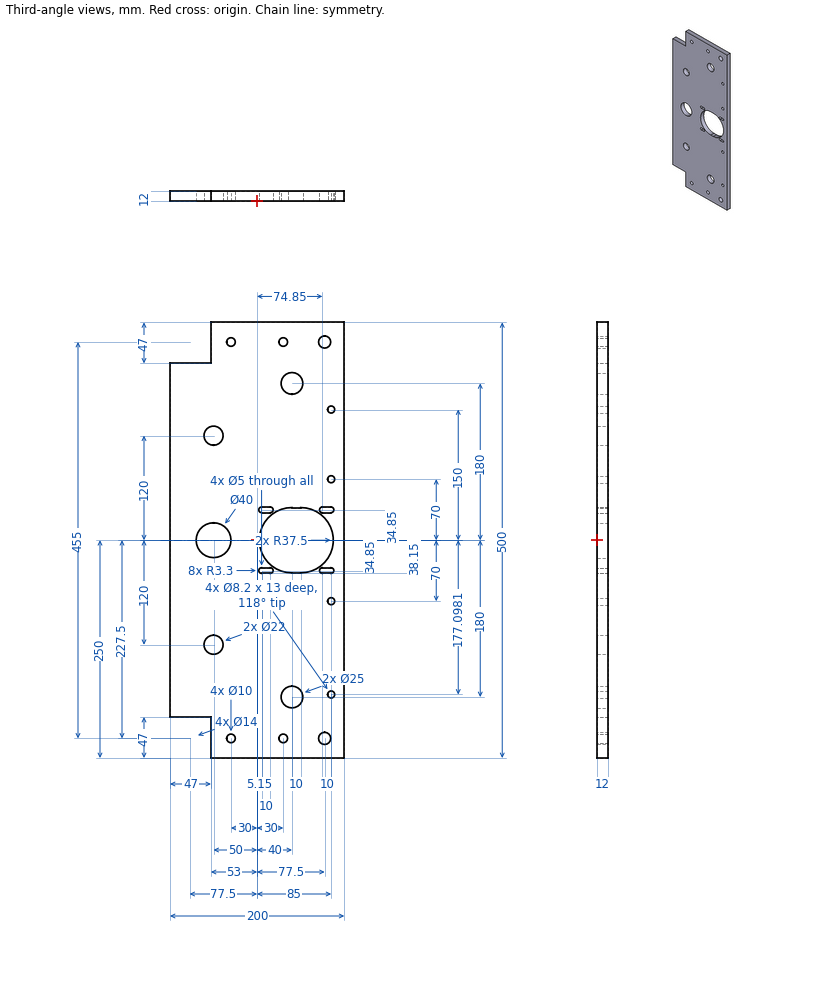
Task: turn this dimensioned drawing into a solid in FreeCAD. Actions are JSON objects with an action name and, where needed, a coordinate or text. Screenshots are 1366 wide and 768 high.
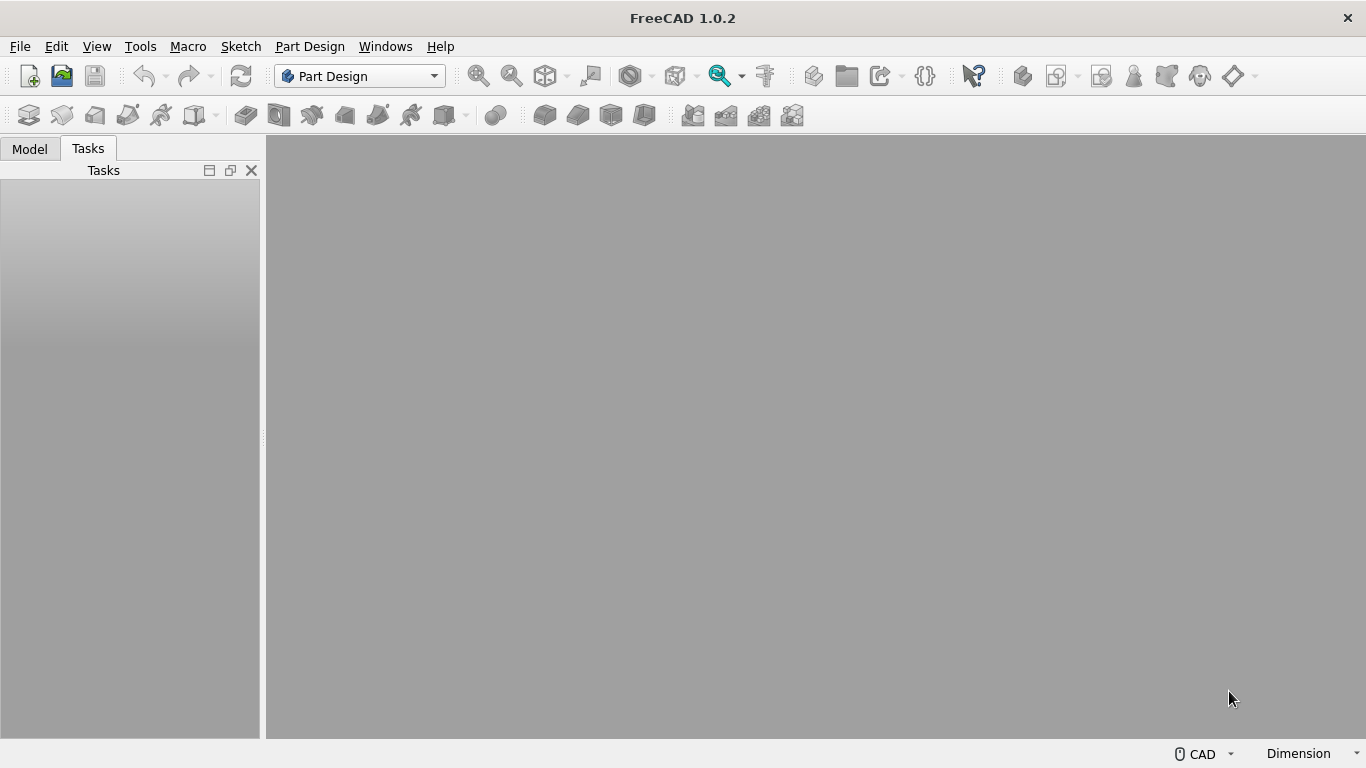
{"action": "key", "text": "ctrl+n"}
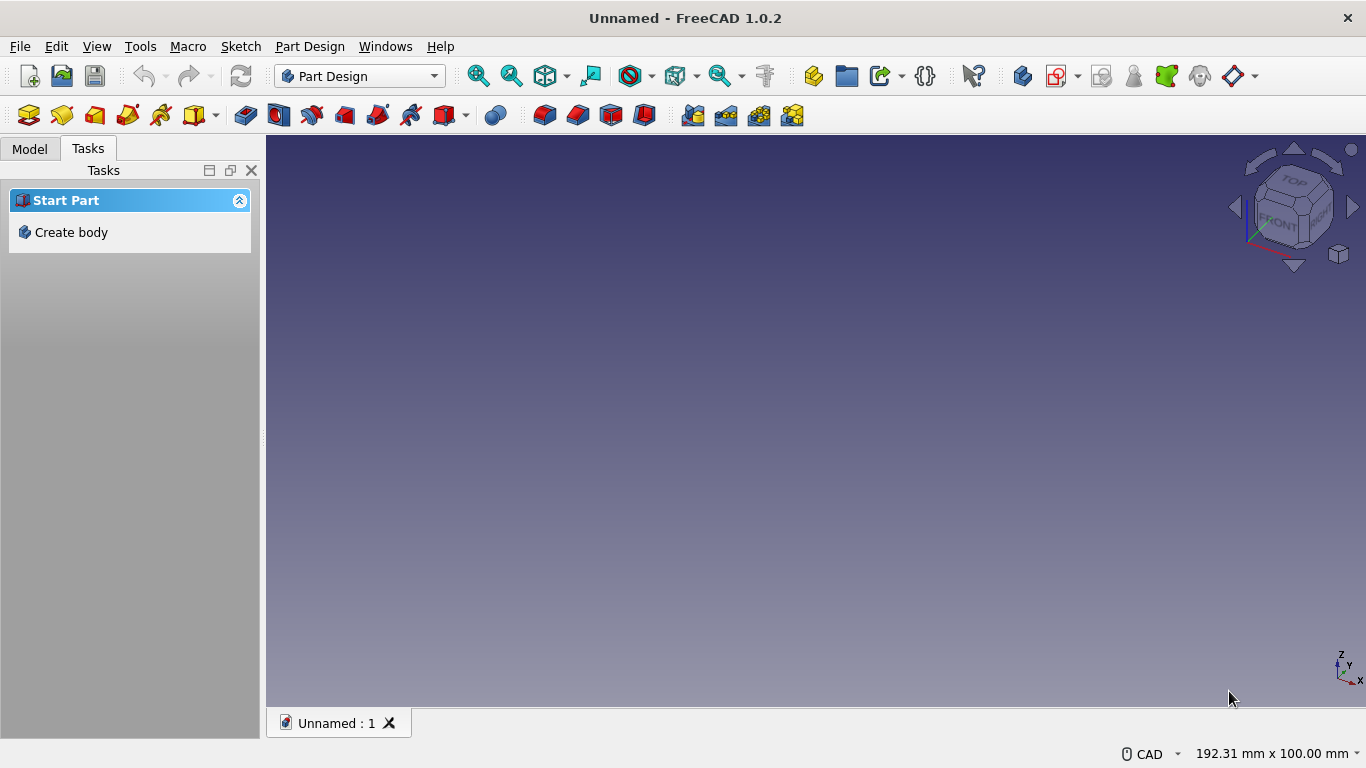
{"action": "left_click", "coordinate": [1056, 76]}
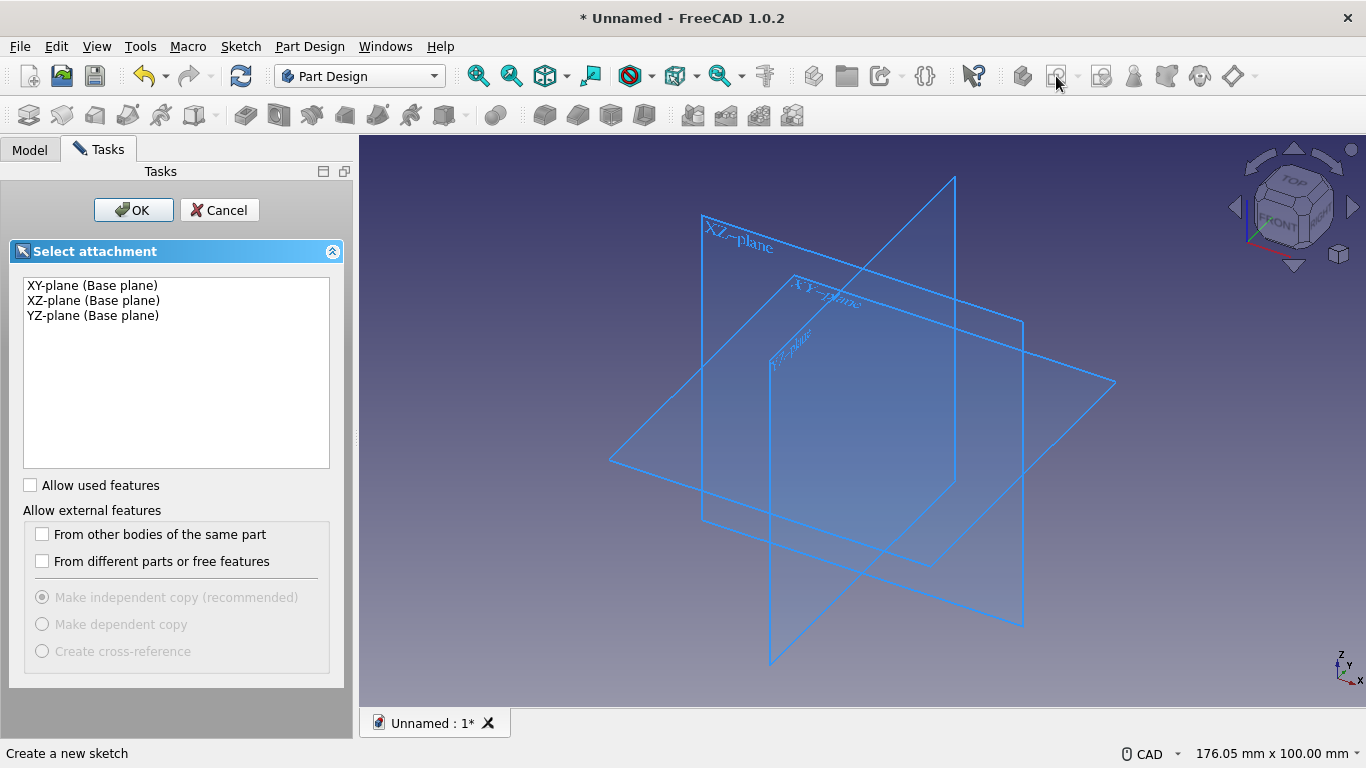
{"action": "left_click", "coordinate": [84, 300]}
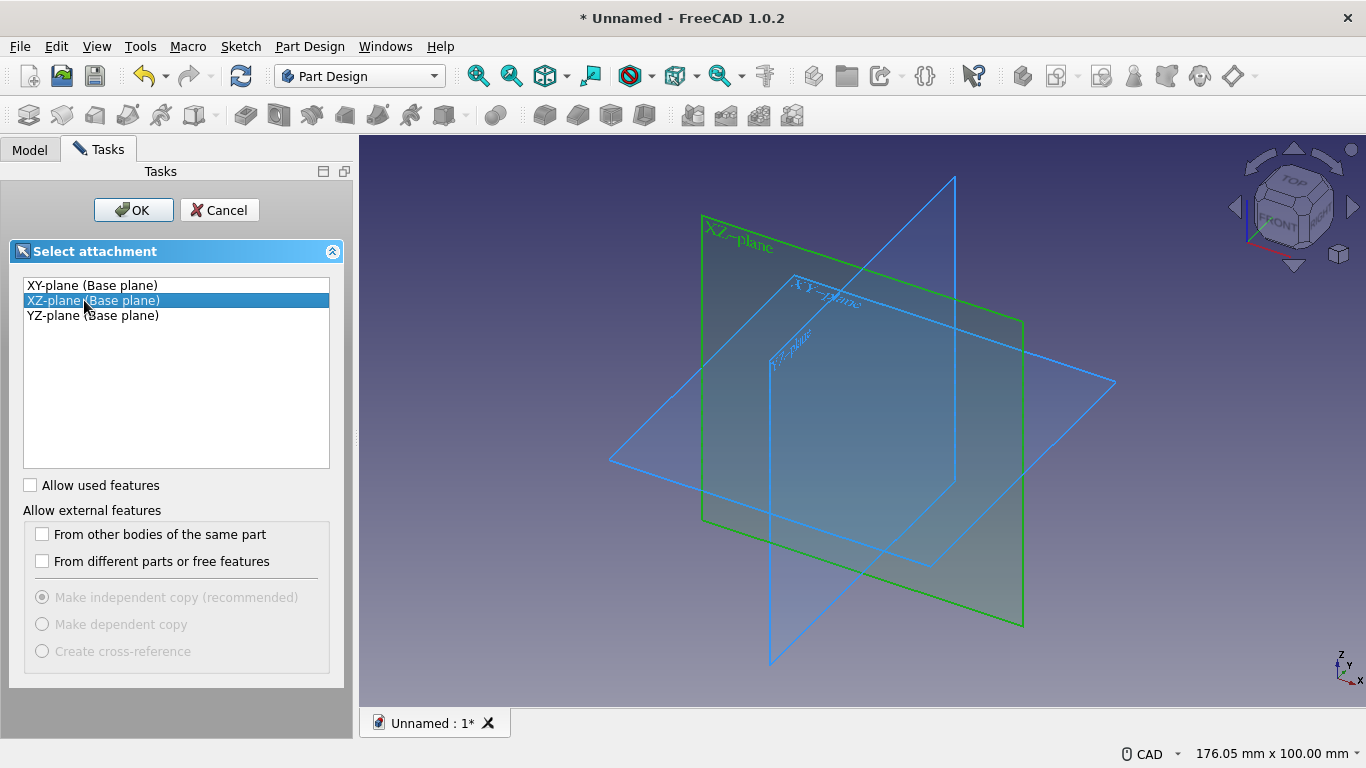
{"action": "left_click", "coordinate": [134, 210]}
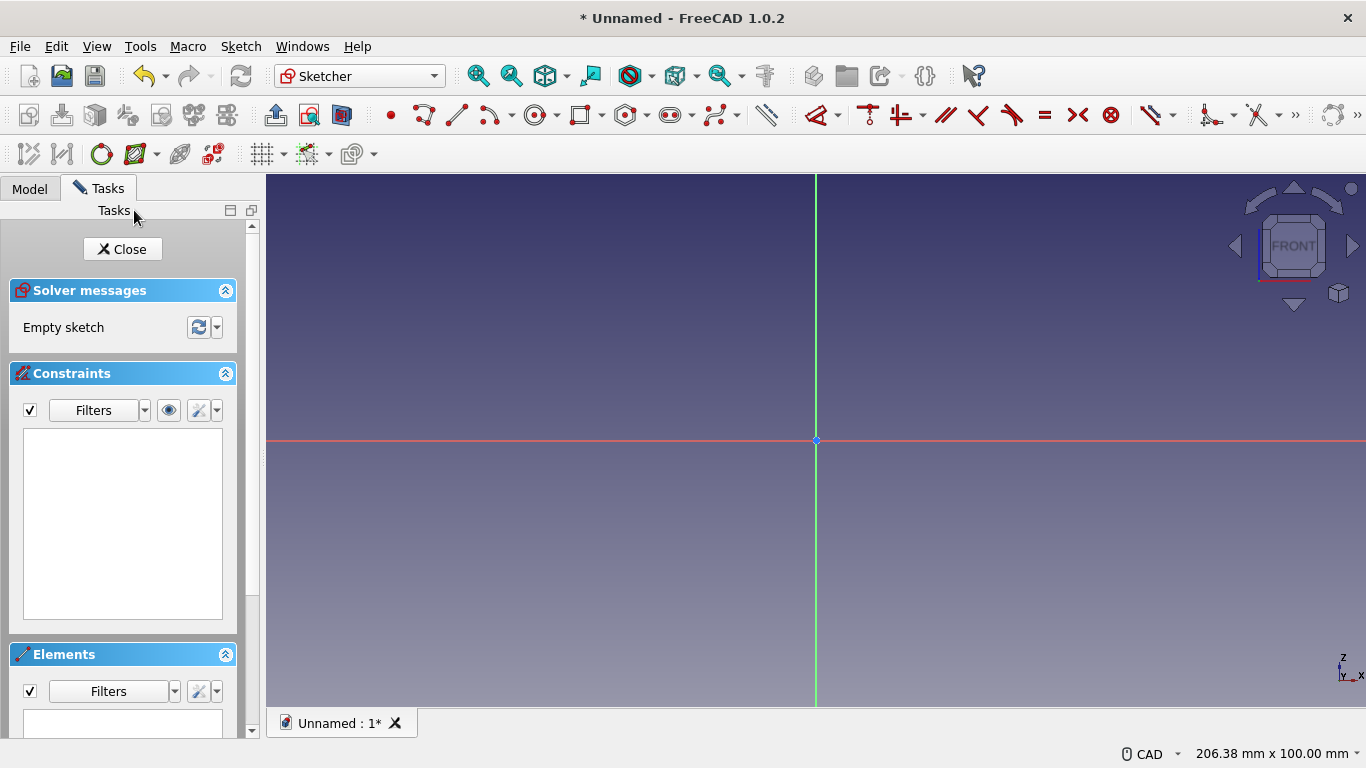
{"action": "scroll", "coordinate": [737, 440], "scroll_direction": "down", "scroll_amount": 10}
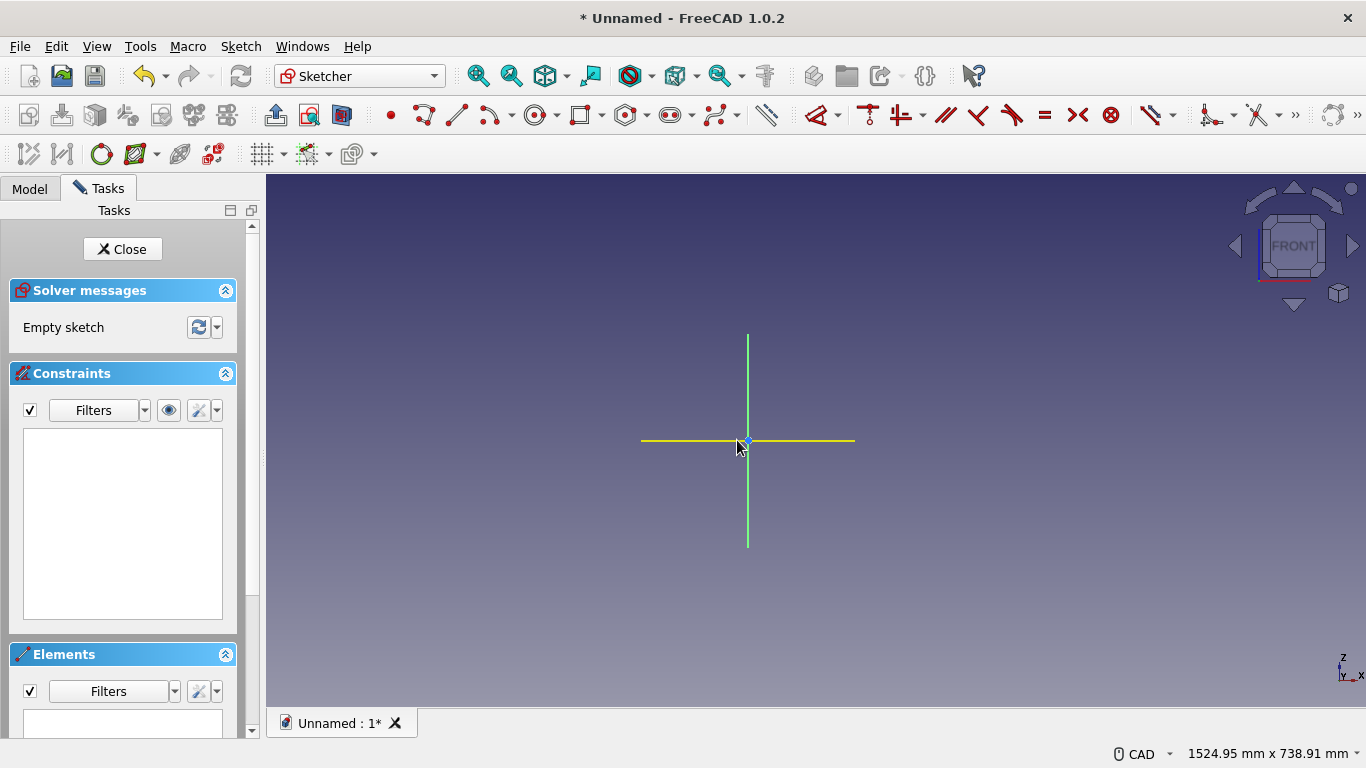
{"action": "key", "text": "g v"}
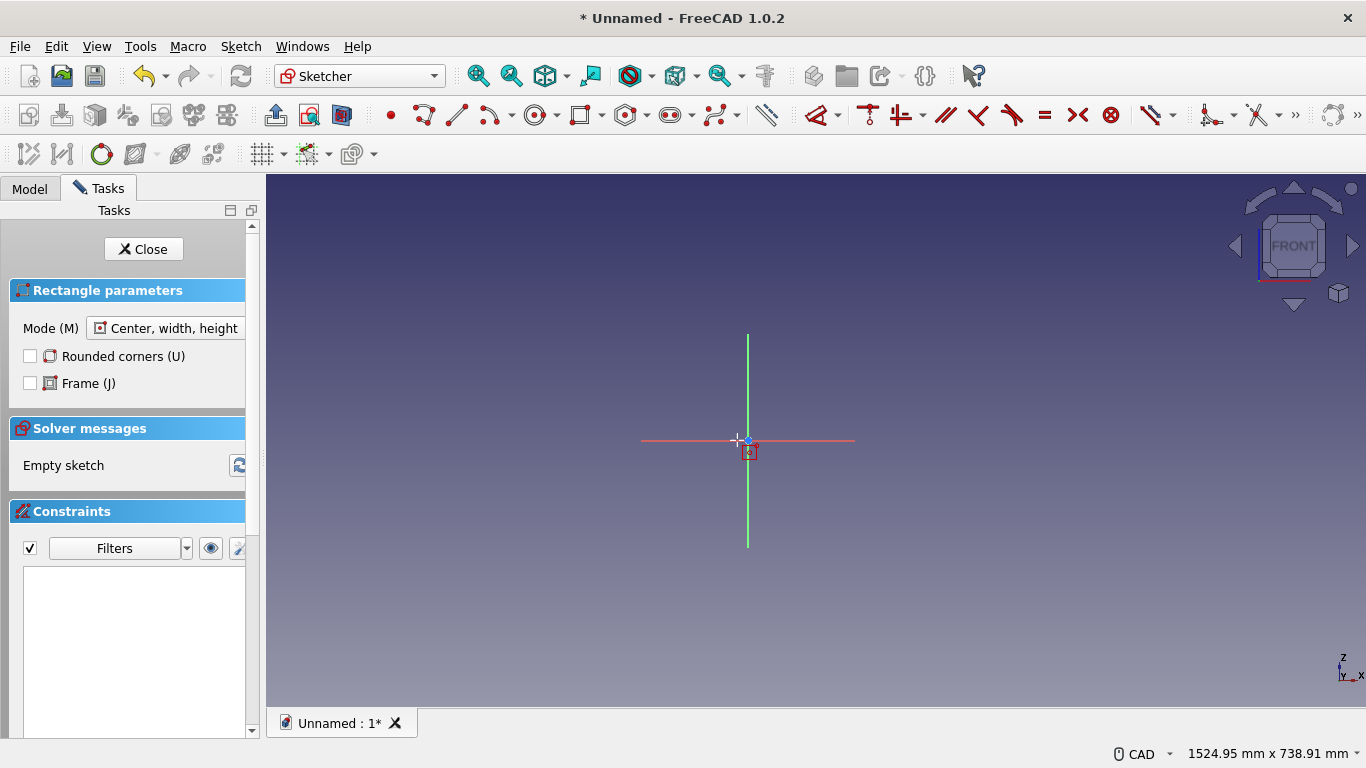
{"action": "left_click", "coordinate": [748, 440]}
{"action": "mouse_move", "coordinate": [820, 260]}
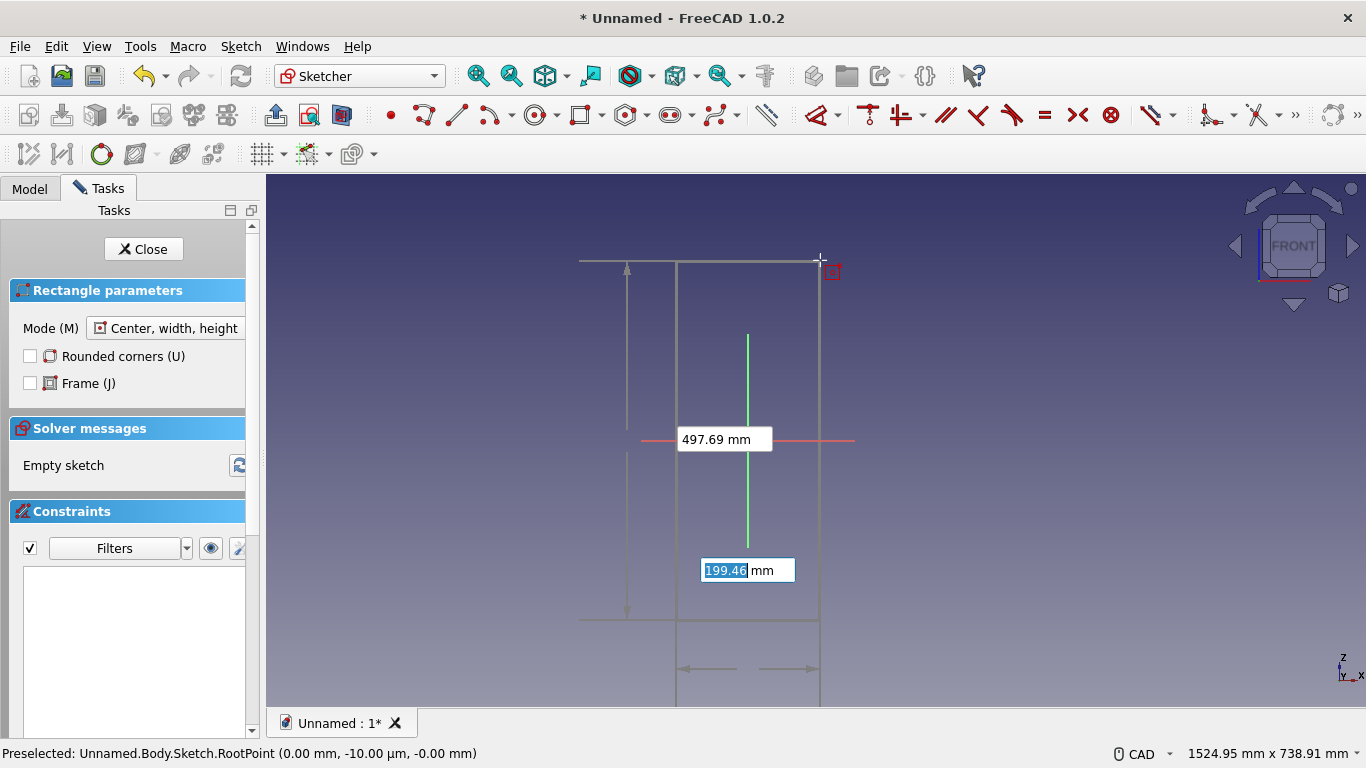
{"action": "type", "text": "200"}
{"action": "key", "text": "Tab"}
{"action": "type", "text": "500"}
{"action": "key", "text": "Return"}
{"action": "key", "text": "Escape"}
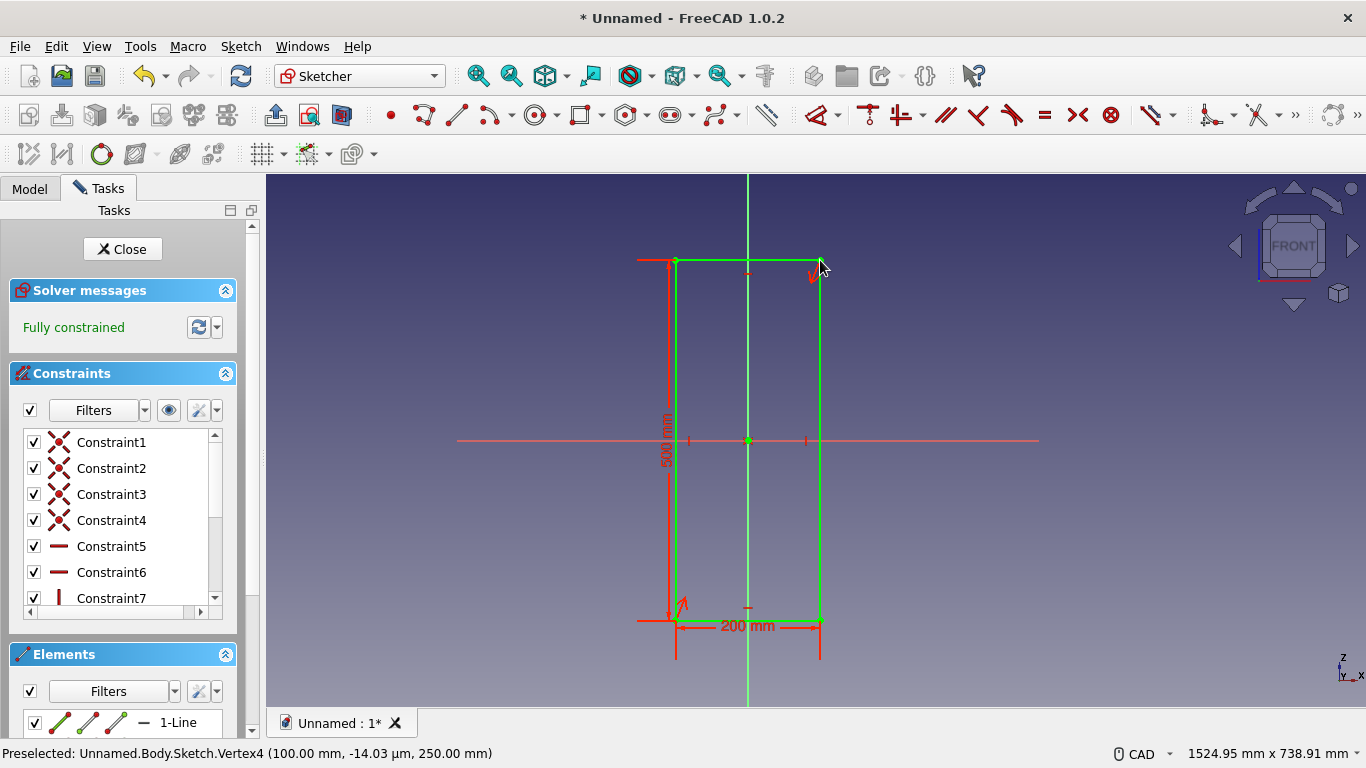
{"action": "left_click", "coordinate": [123, 249]}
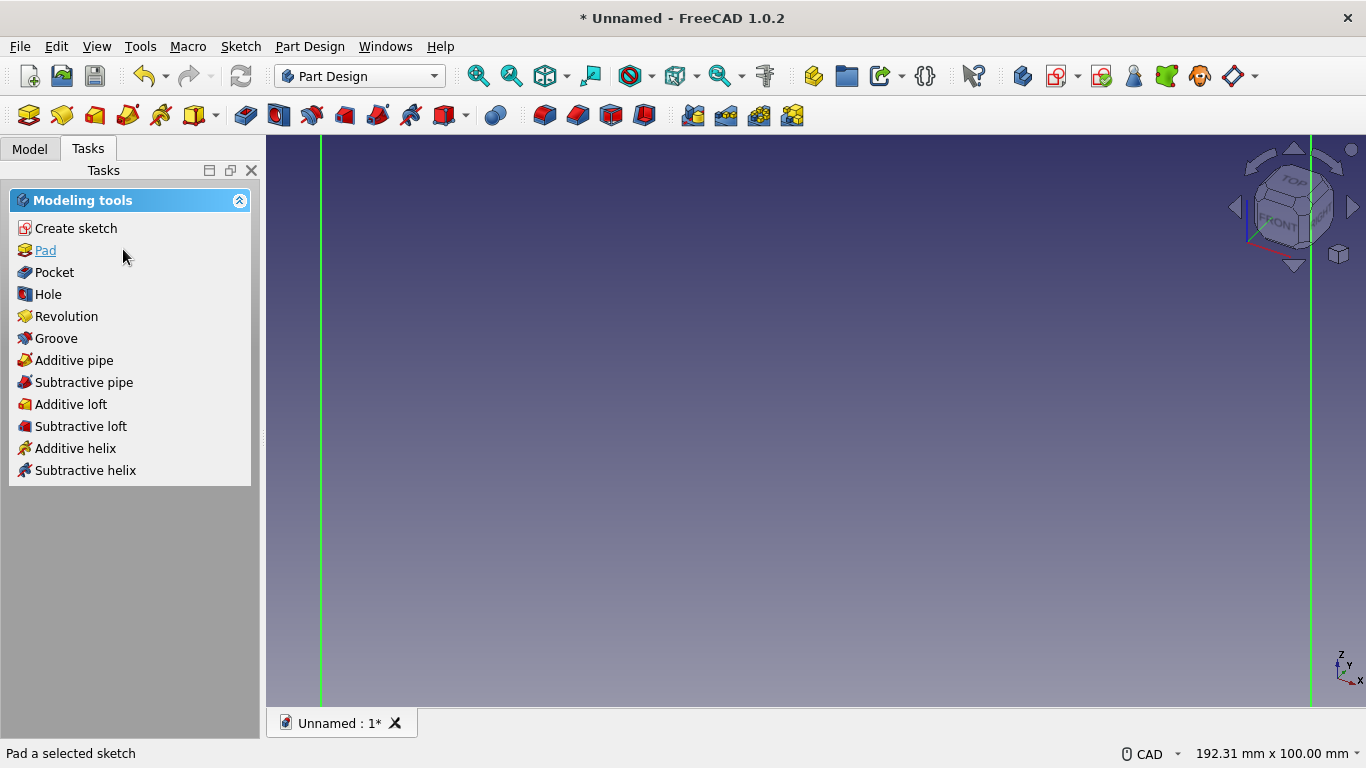
{"action": "left_click", "coordinate": [29, 116]}